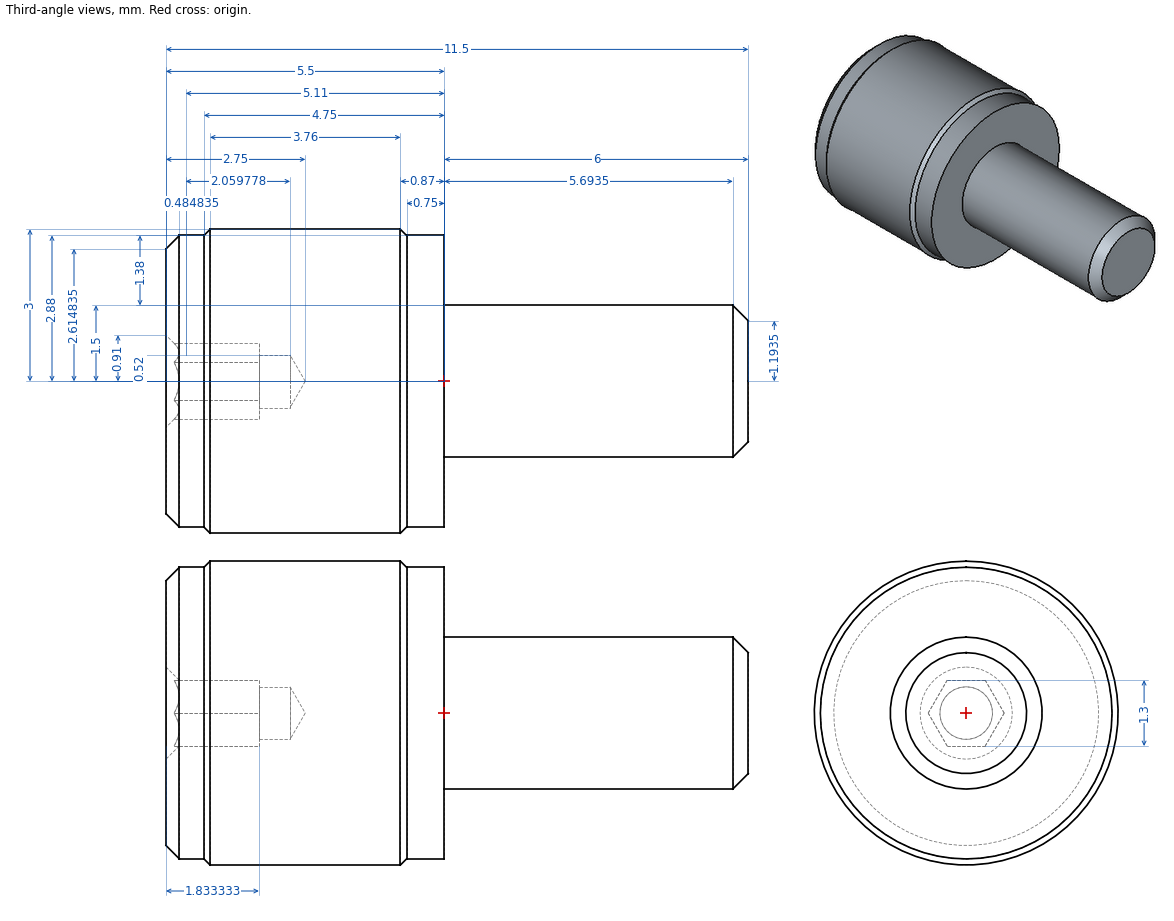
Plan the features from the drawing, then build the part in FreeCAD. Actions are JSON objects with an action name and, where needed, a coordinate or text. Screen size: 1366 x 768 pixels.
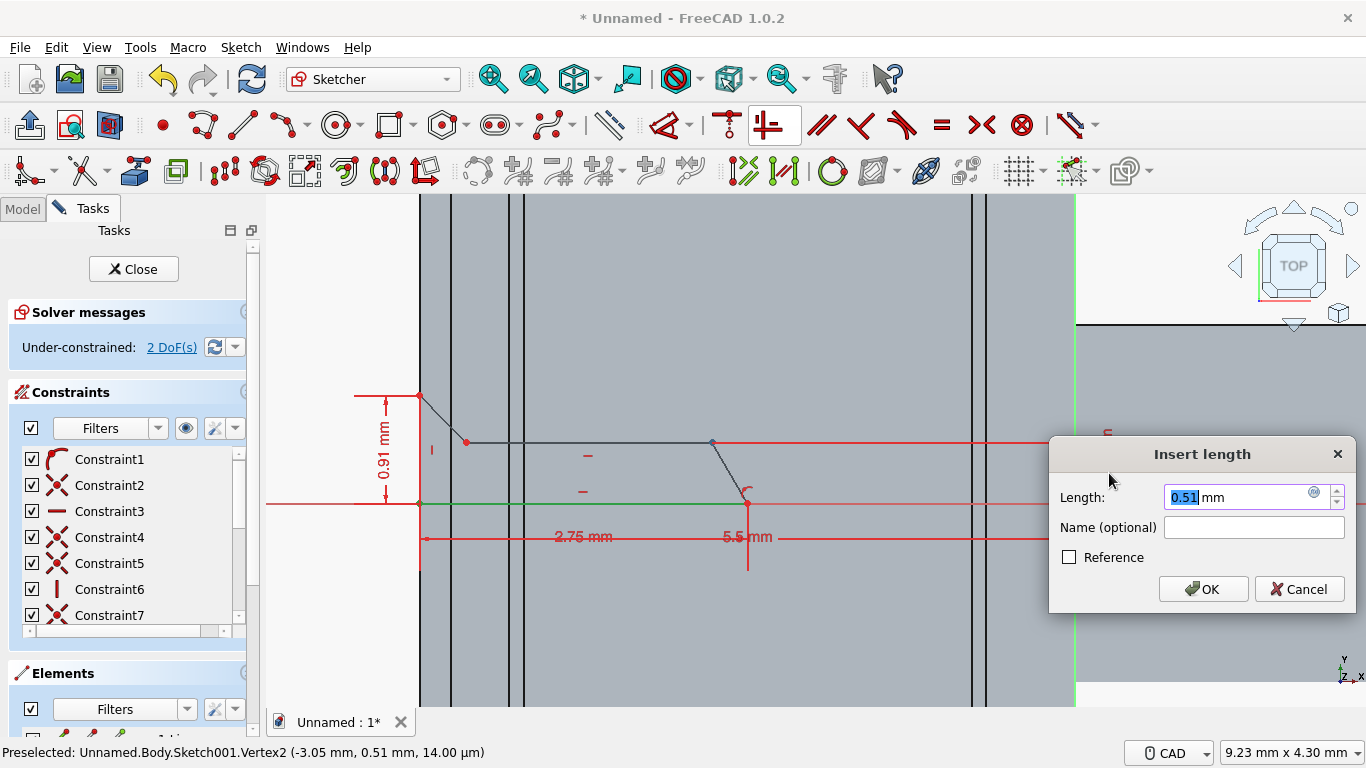
{"action": "type", "text": "0.52"}
{"action": "key", "text": "Return"}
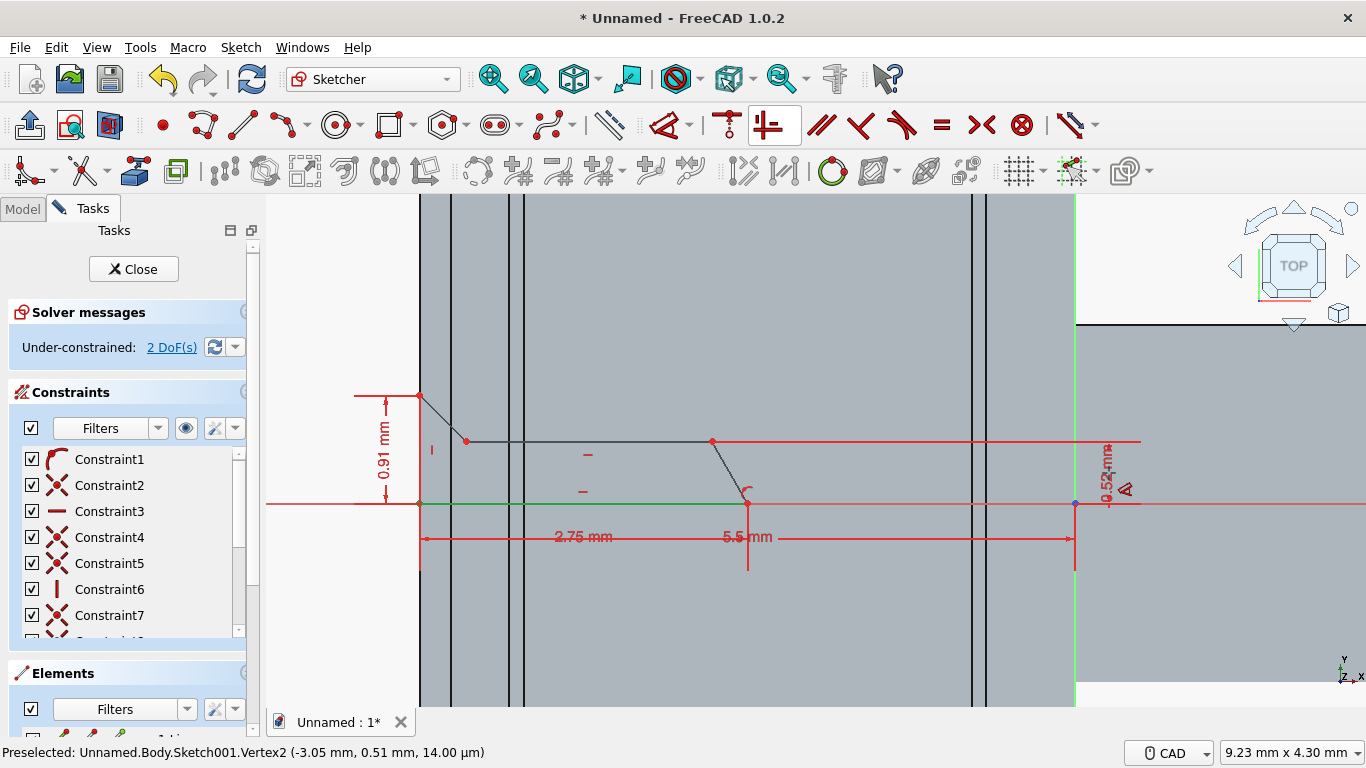
{"action": "left_click", "coordinate": [466, 442]}
{"action": "left_click", "coordinate": [911, 538]}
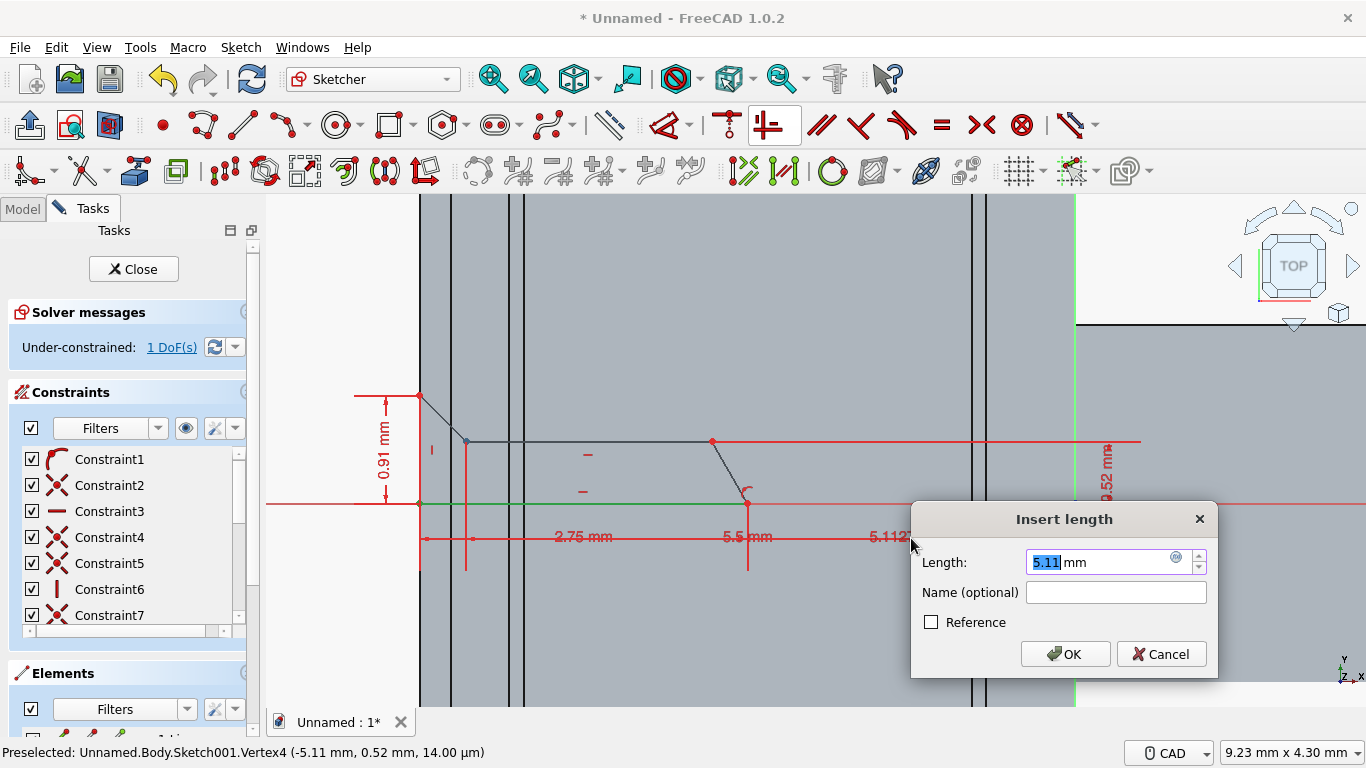
{"action": "type", "text": "5.11"}
{"action": "key", "text": "Return"}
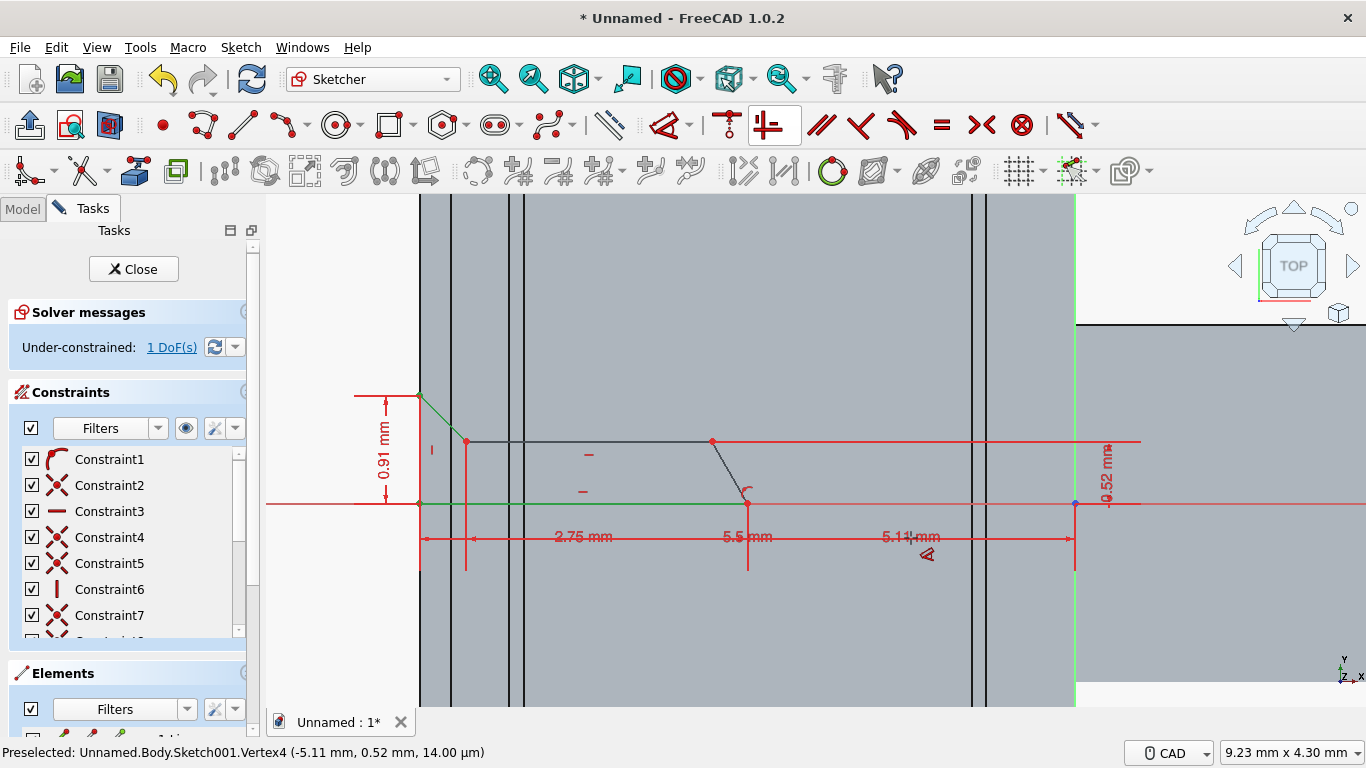
{"action": "left_click", "coordinate": [638, 442]}
{"action": "left_click", "coordinate": [589, 408]}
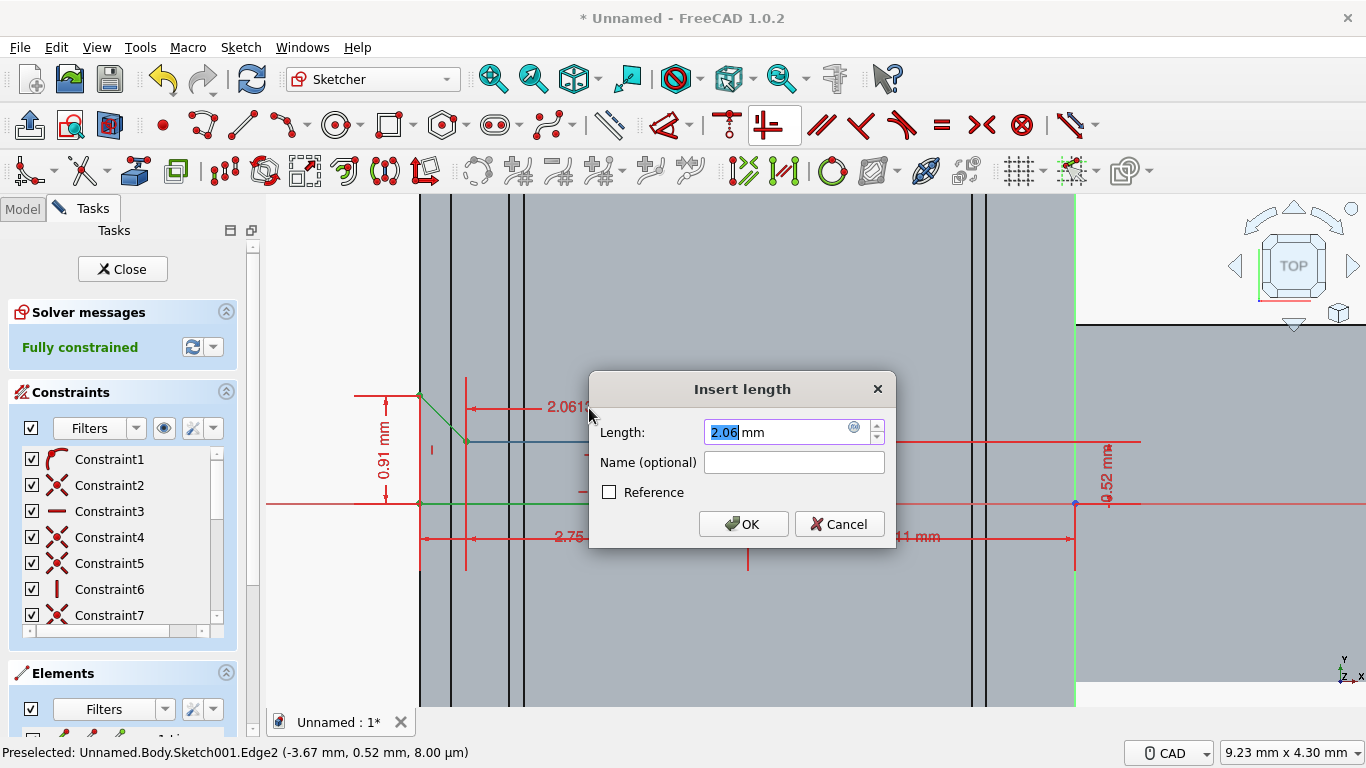
{"action": "type", "text": "2.059778"}
{"action": "key", "text": "Return"}
{"action": "key", "text": "Escape"}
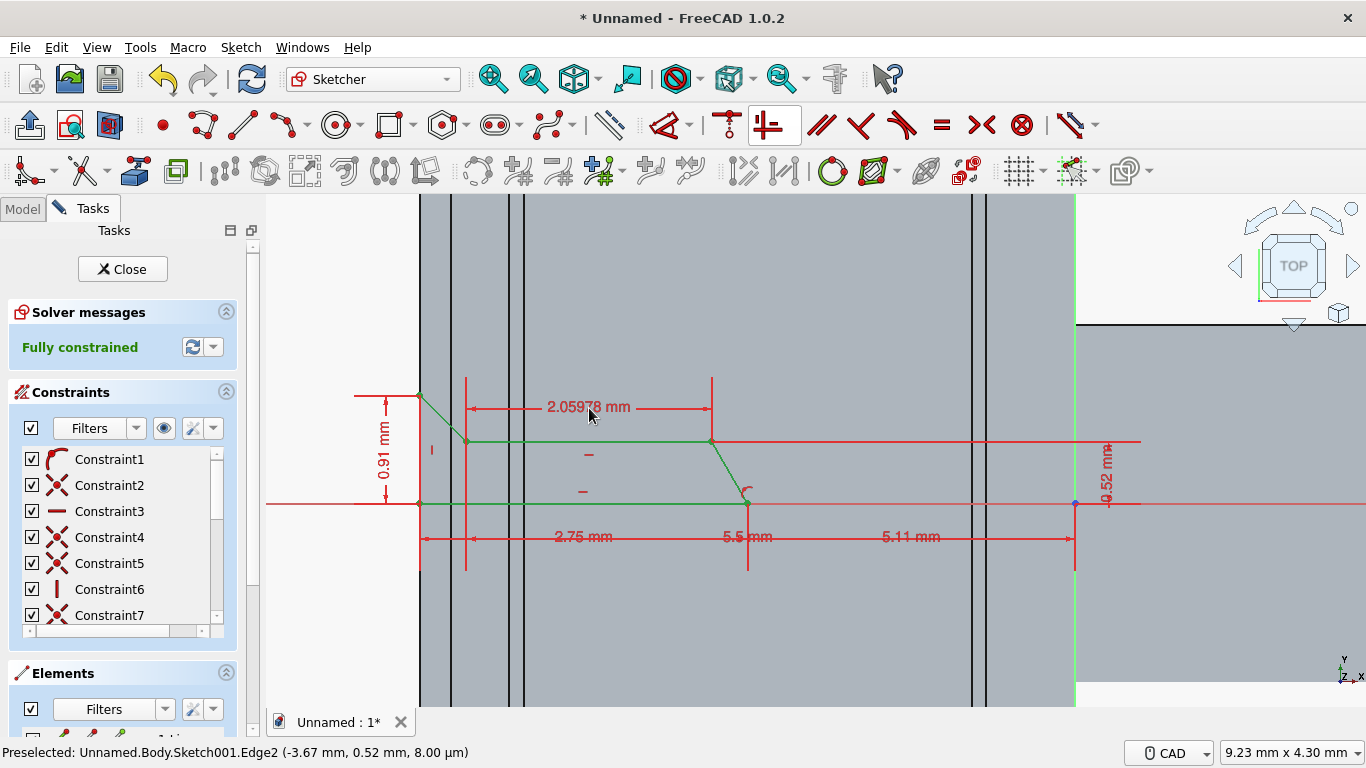
{"action": "left_click", "coordinate": [123, 269]}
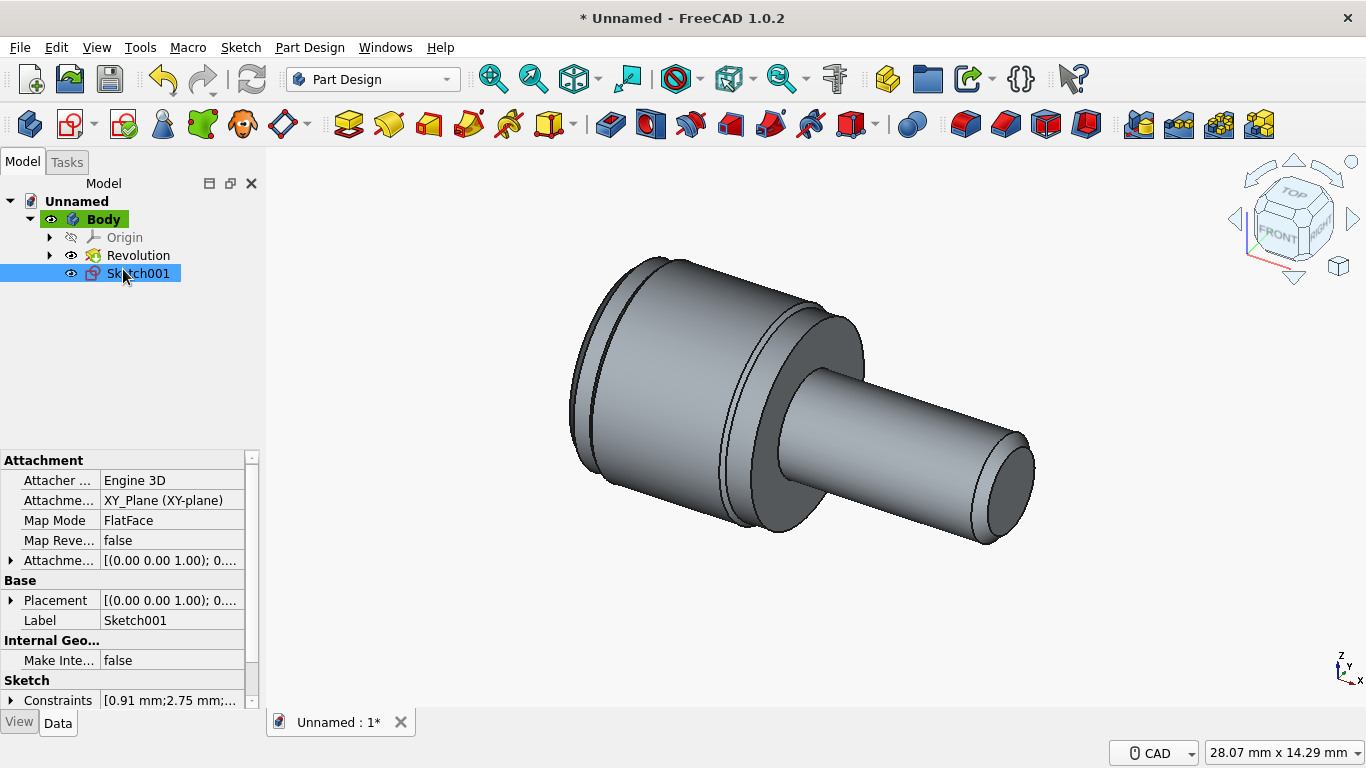
{"action": "left_click", "coordinate": [692, 124]}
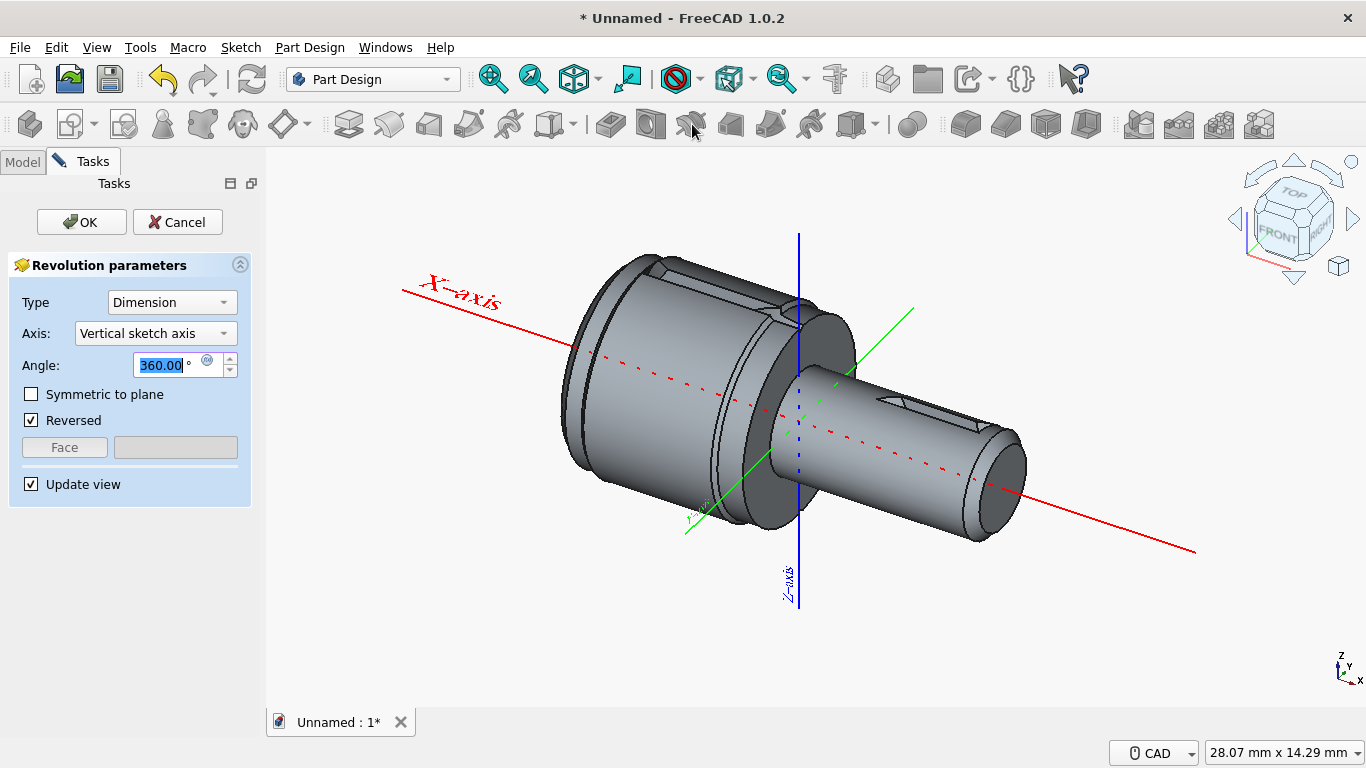
{"action": "left_click", "coordinate": [156, 334]}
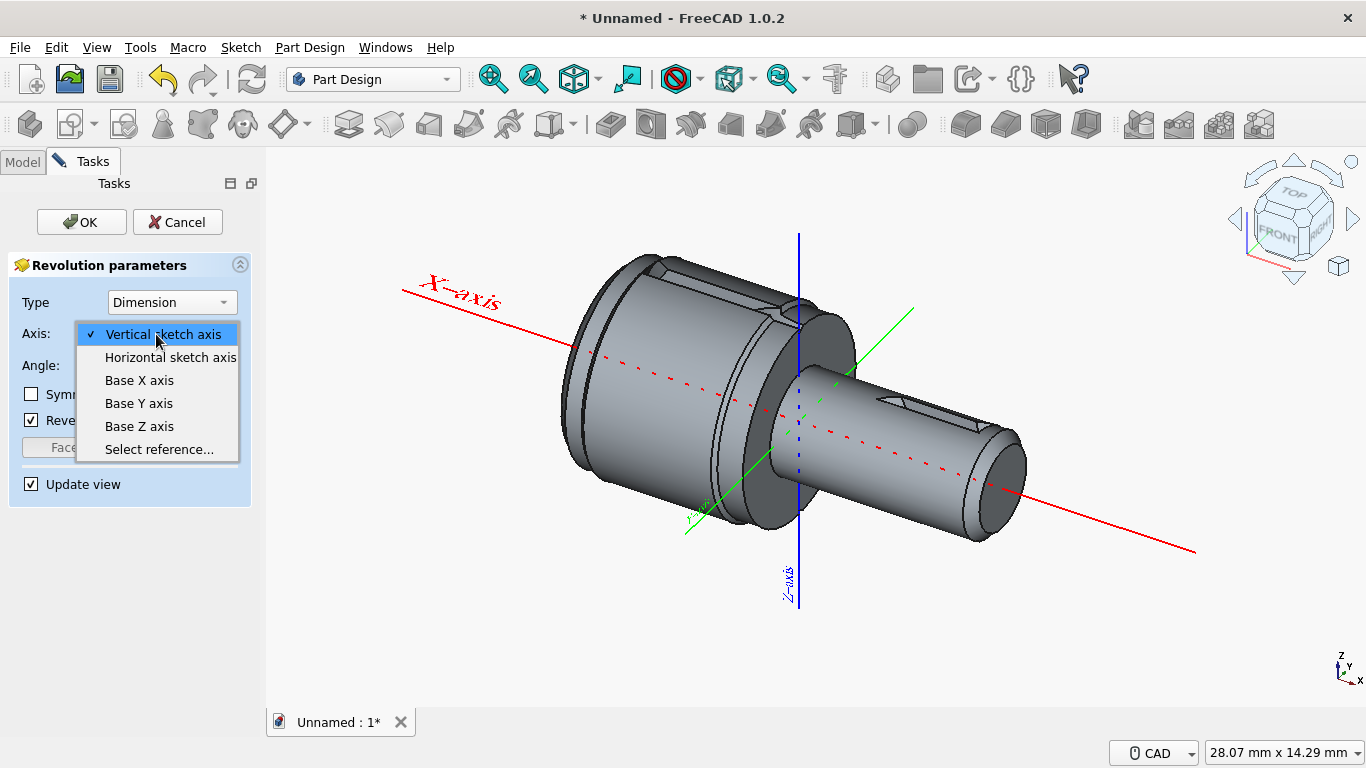
{"action": "left_click", "coordinate": [156, 358]}